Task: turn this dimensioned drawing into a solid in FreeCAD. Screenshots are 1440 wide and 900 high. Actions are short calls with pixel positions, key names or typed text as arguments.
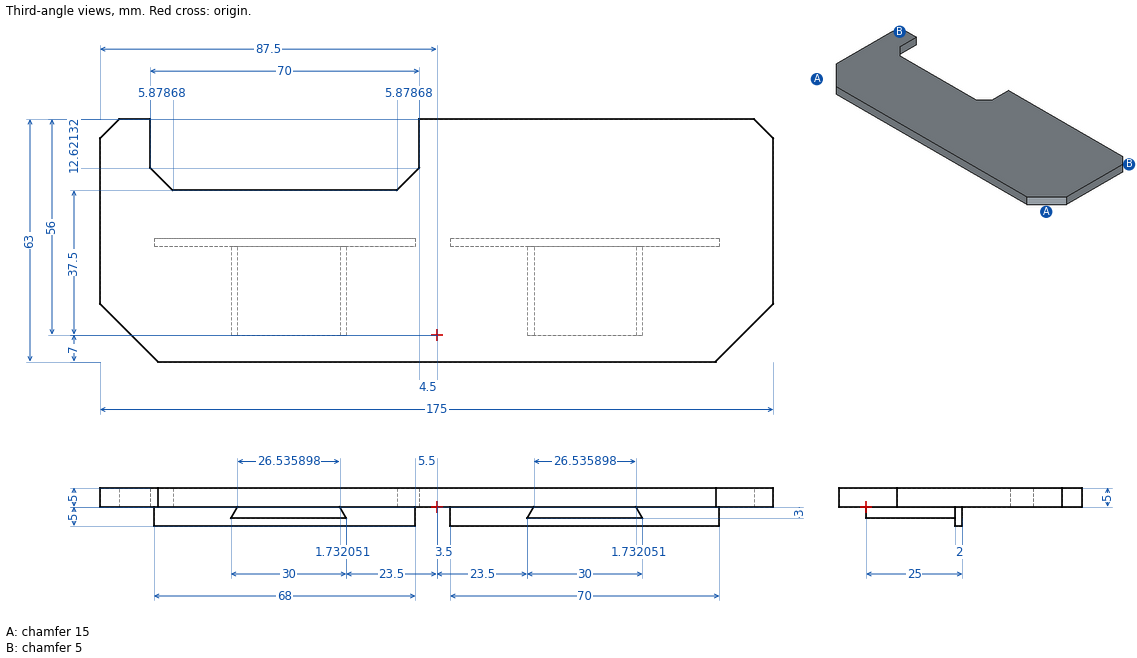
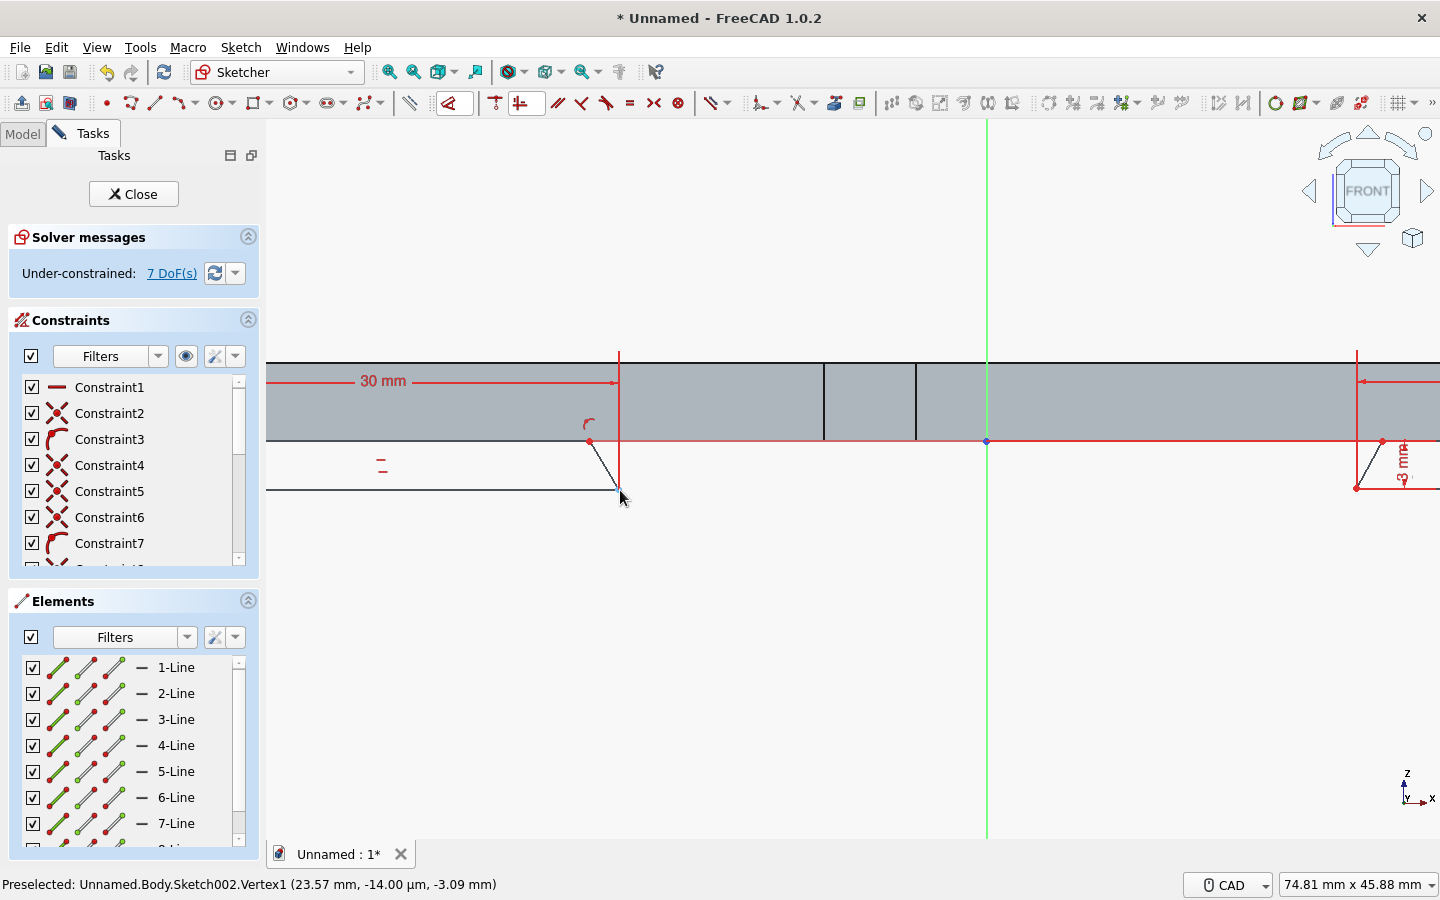
click(619, 490)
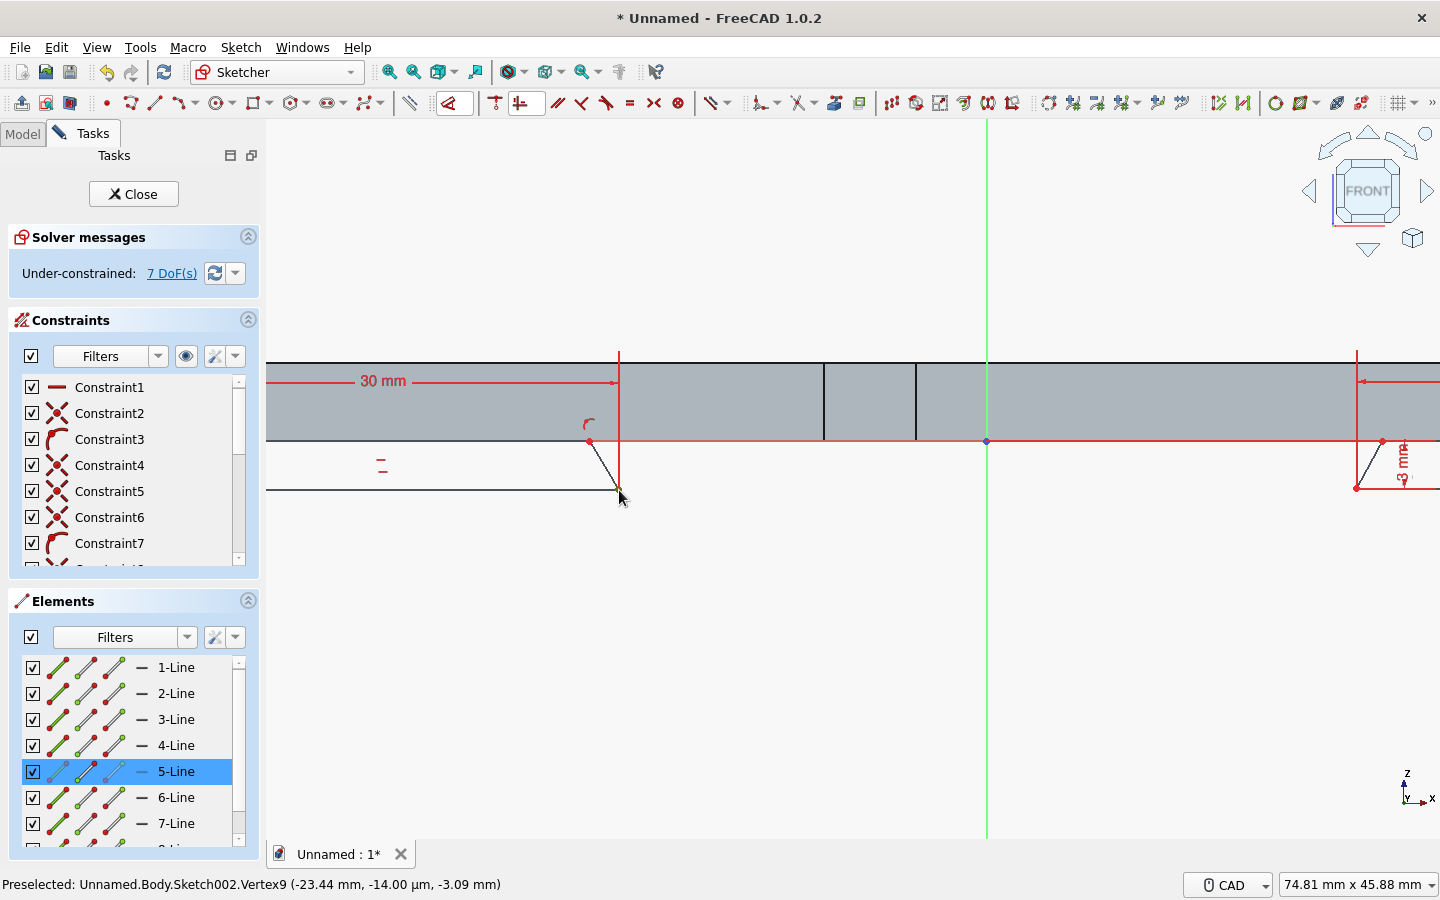
key(i)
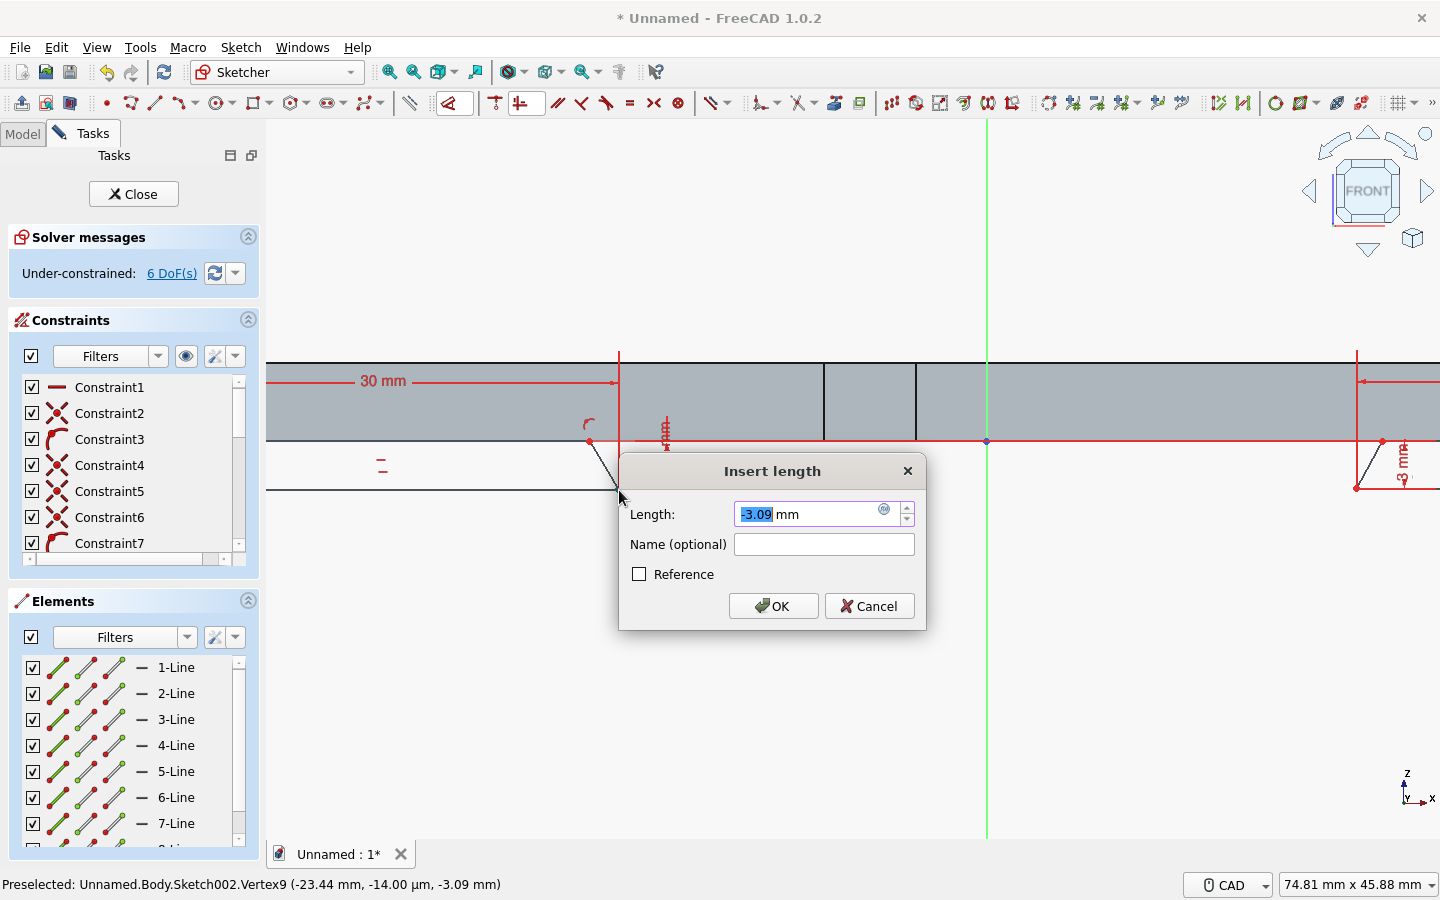
text(-3)
key(Return)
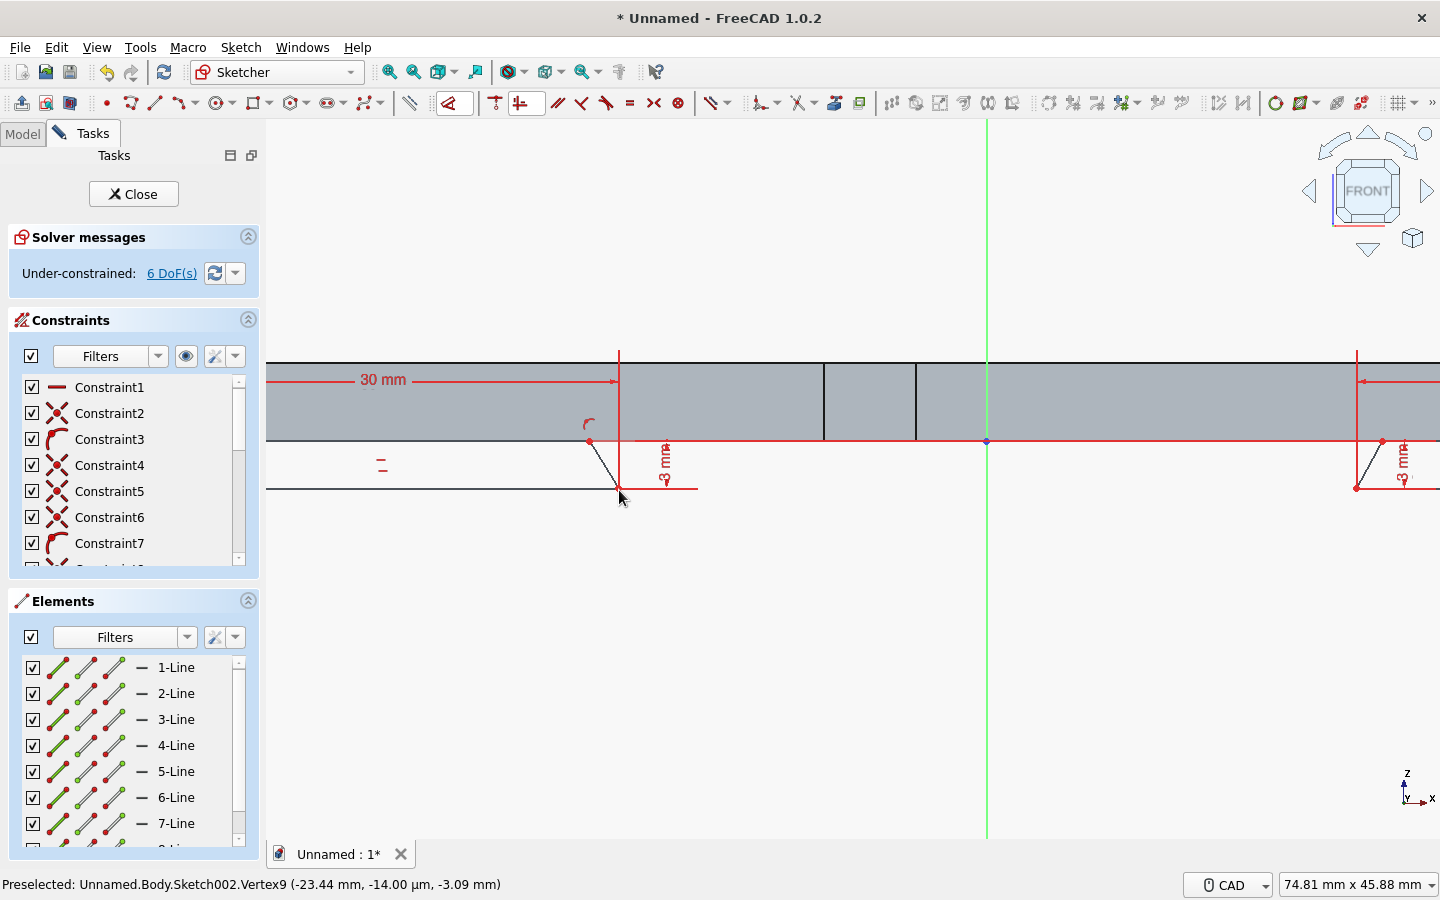
scroll(619, 490, down, 4)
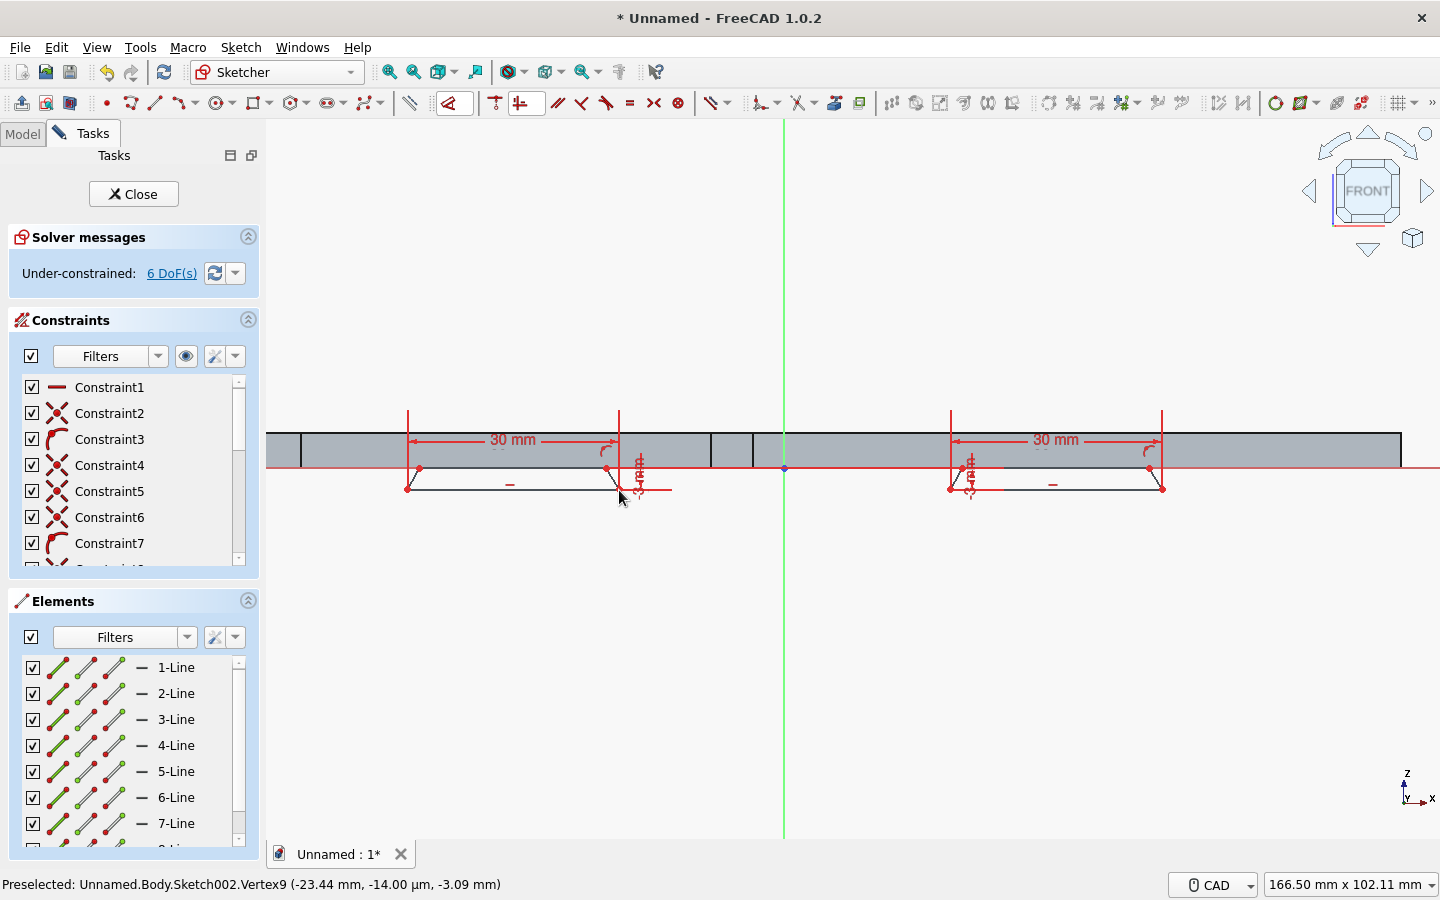
click(951, 490)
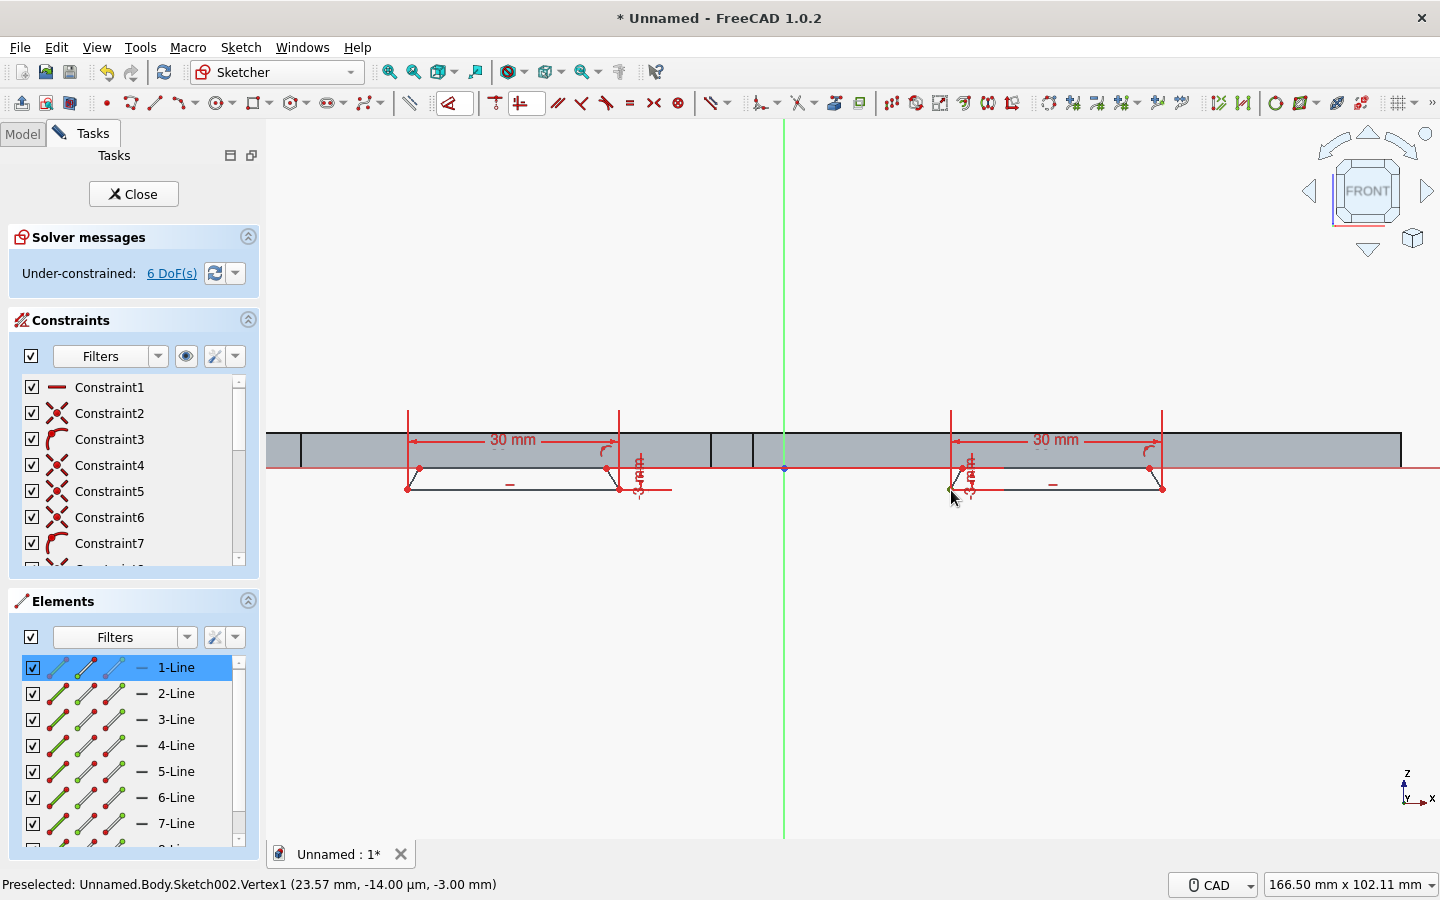
click(468, 104)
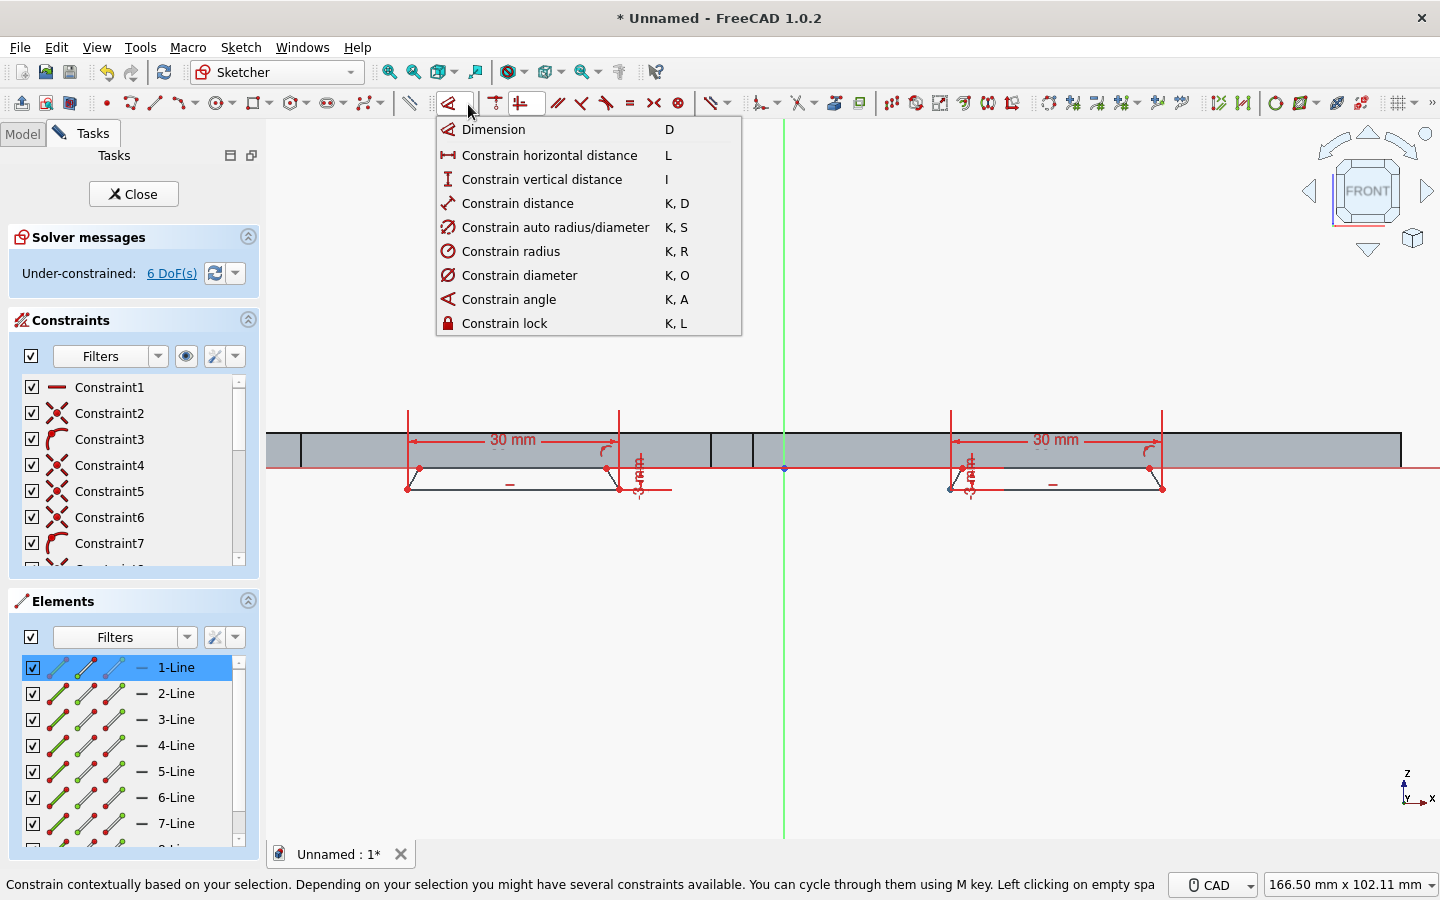
click(589, 155)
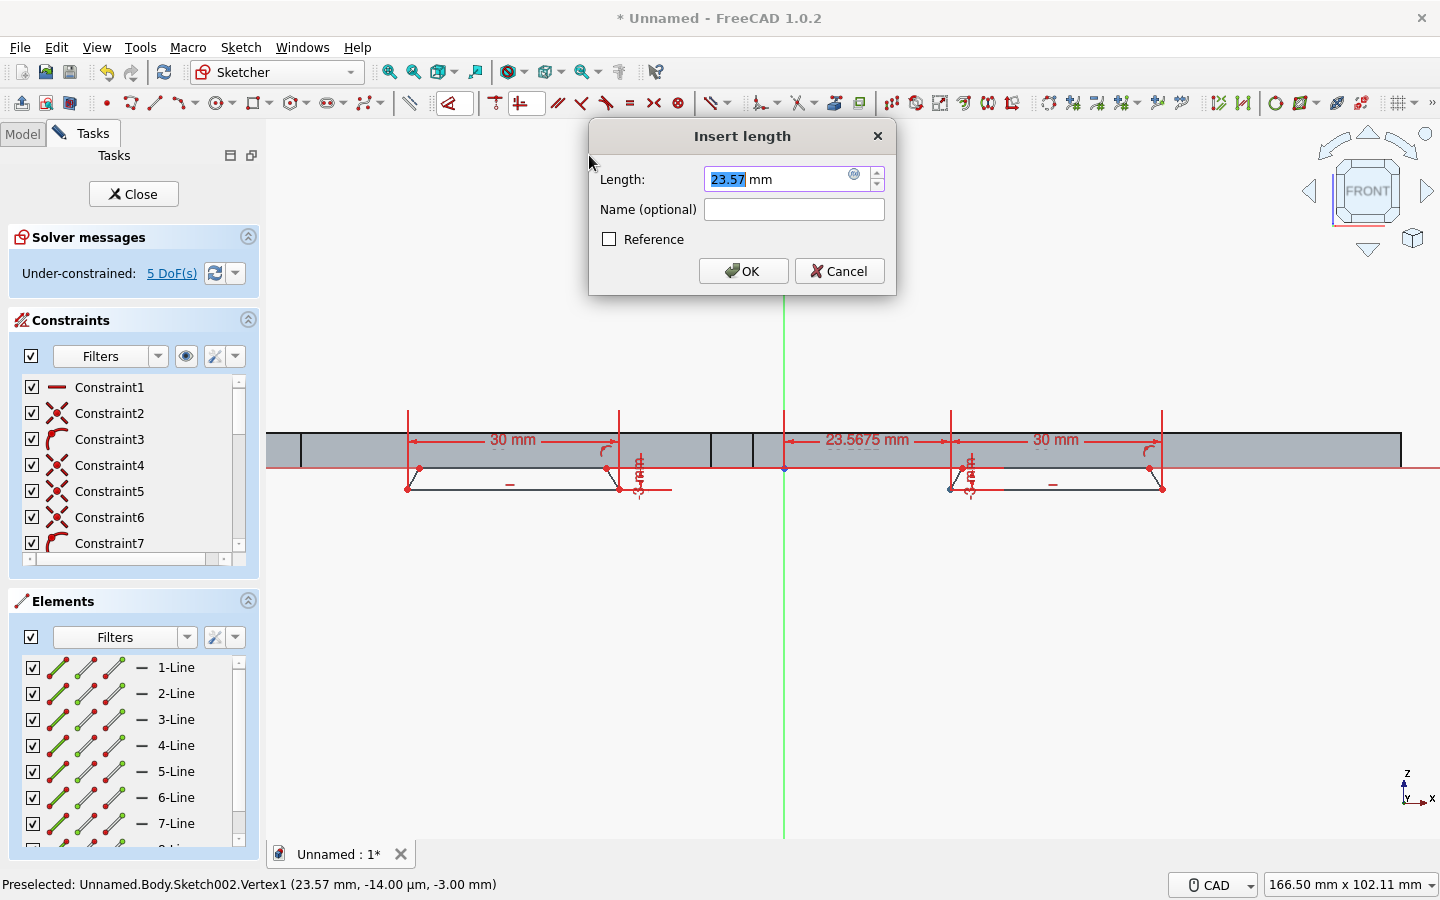
text(23.5)
key(Return)